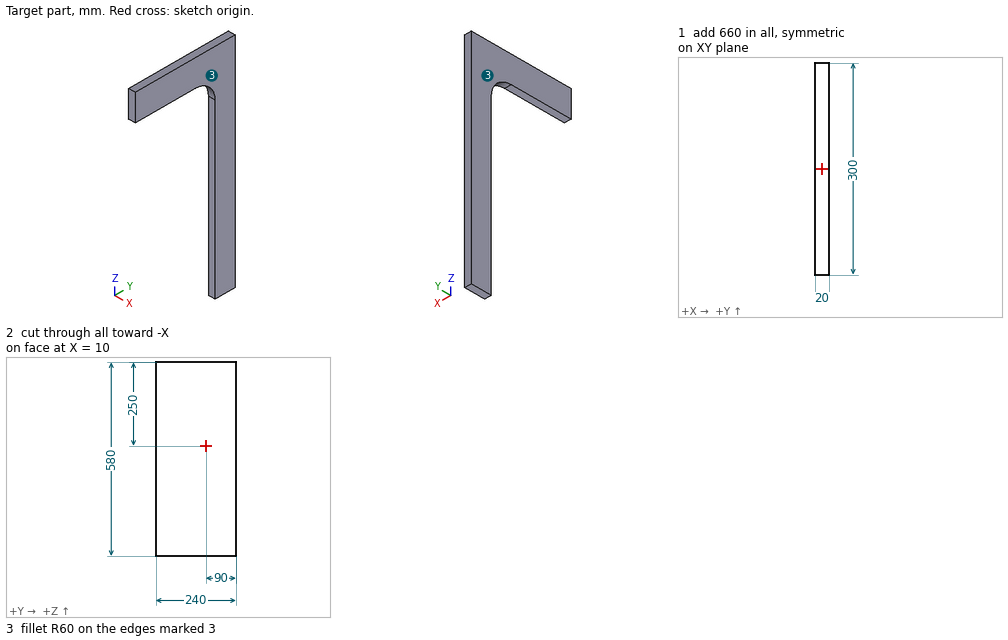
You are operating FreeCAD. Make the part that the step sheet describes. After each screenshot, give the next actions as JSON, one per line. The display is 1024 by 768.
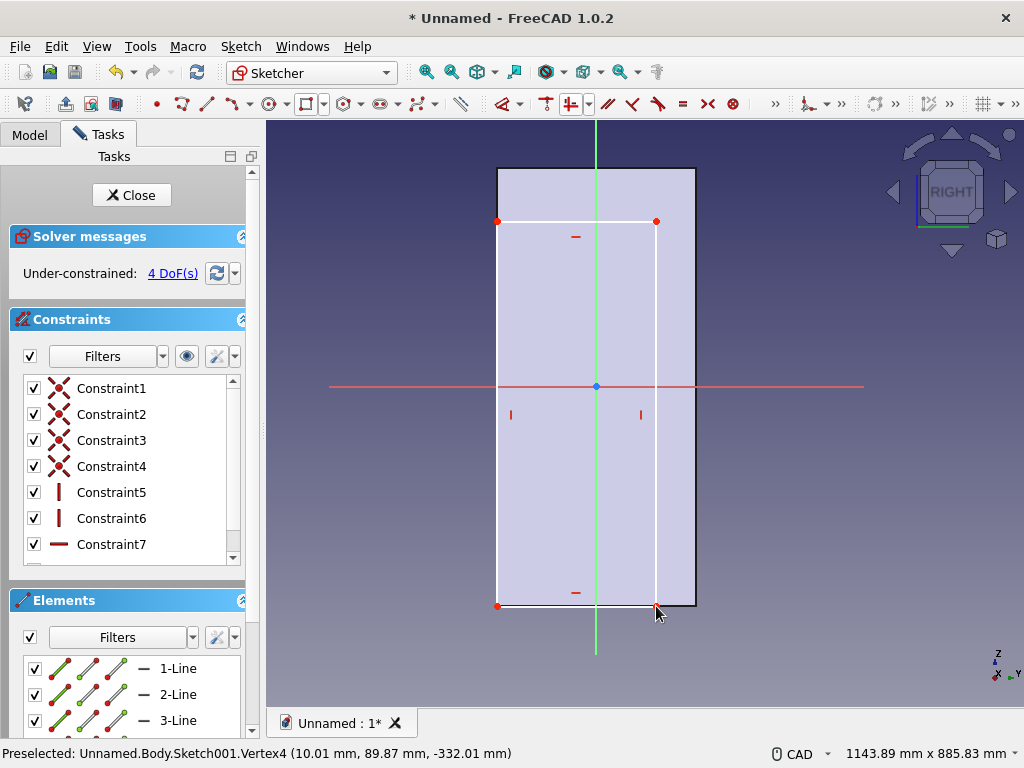
{"action": "key", "text": "d"}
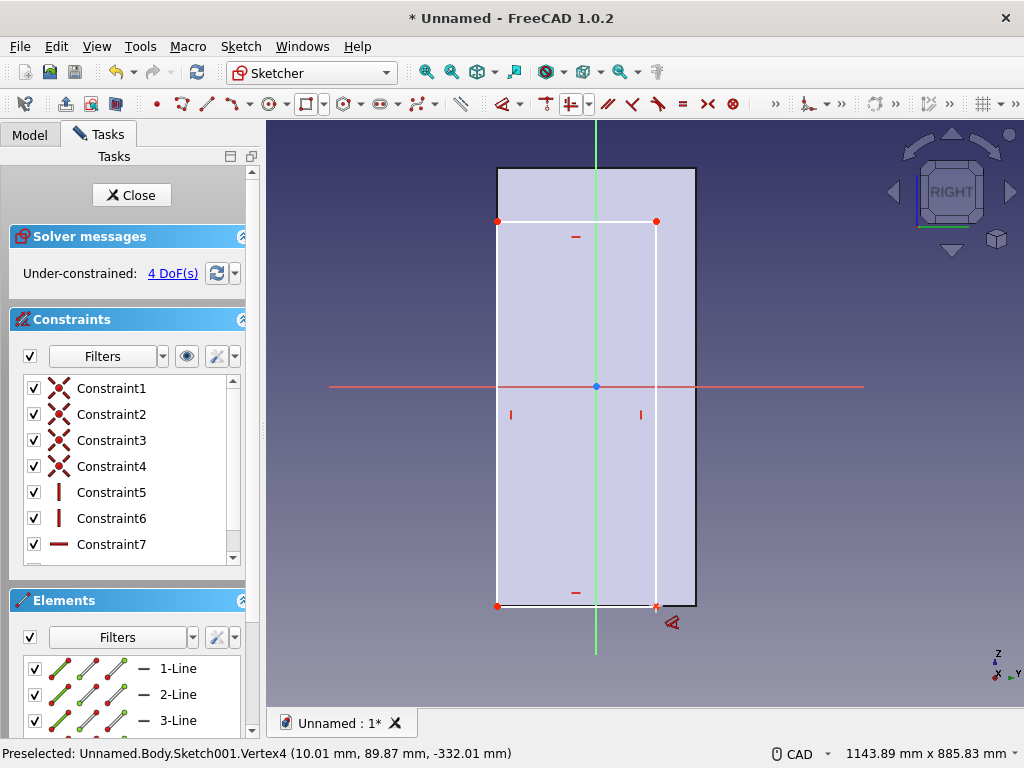
{"action": "left_click", "coordinate": [497, 337]}
{"action": "left_click", "coordinate": [463, 414]}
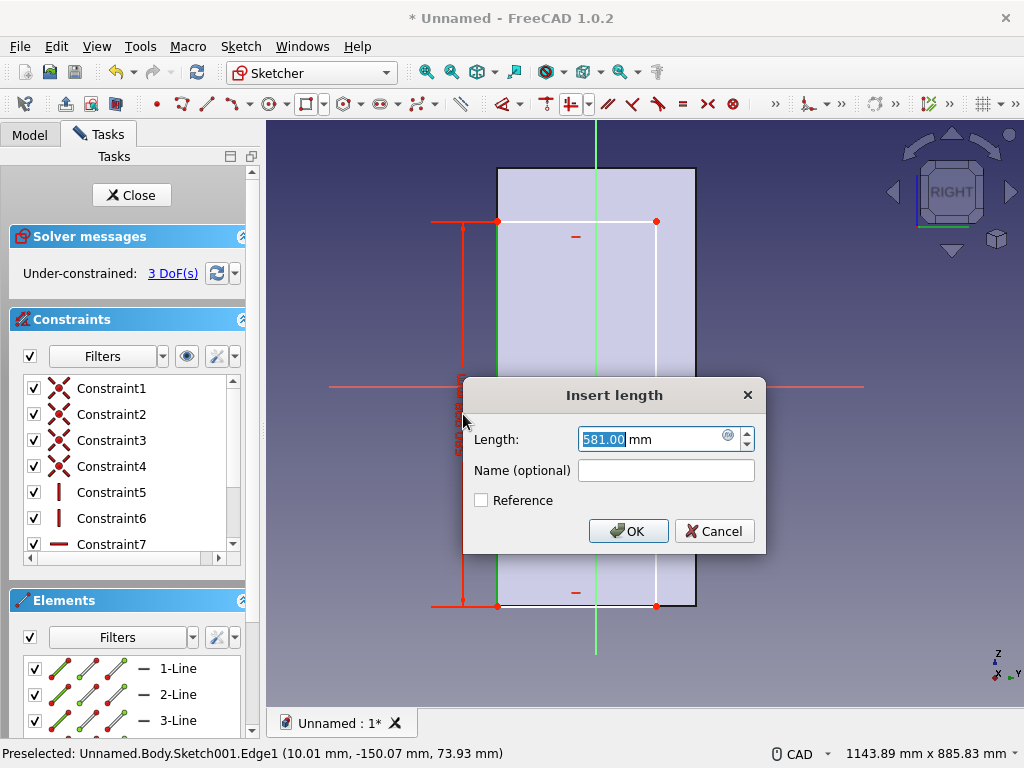
{"action": "type", "text": "580"}
{"action": "key", "text": "Return"}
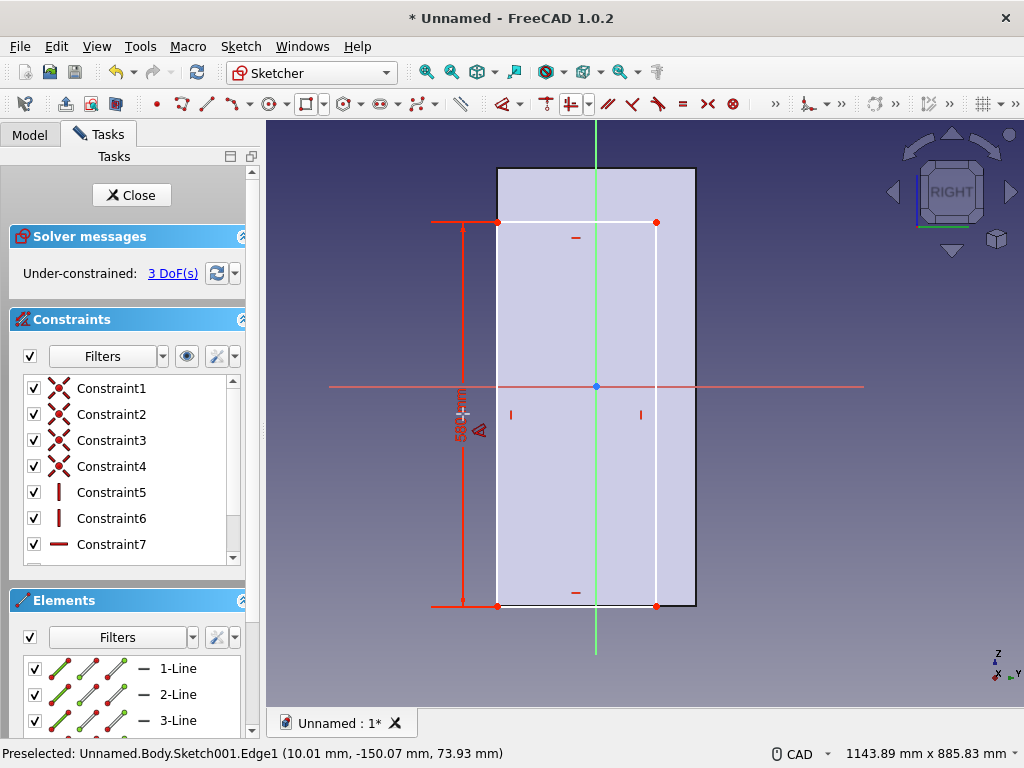
{"action": "left_click", "coordinate": [545, 607]}
{"action": "left_click", "coordinate": [576, 641]}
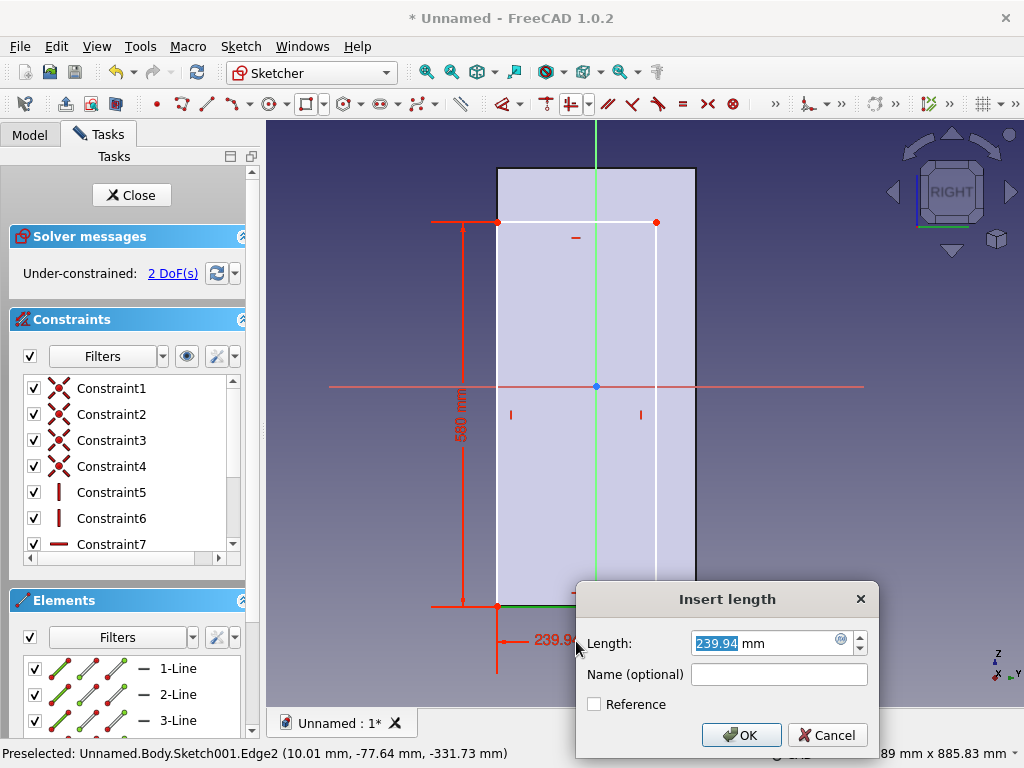
{"action": "type", "text": "240"}
{"action": "key", "text": "Return"}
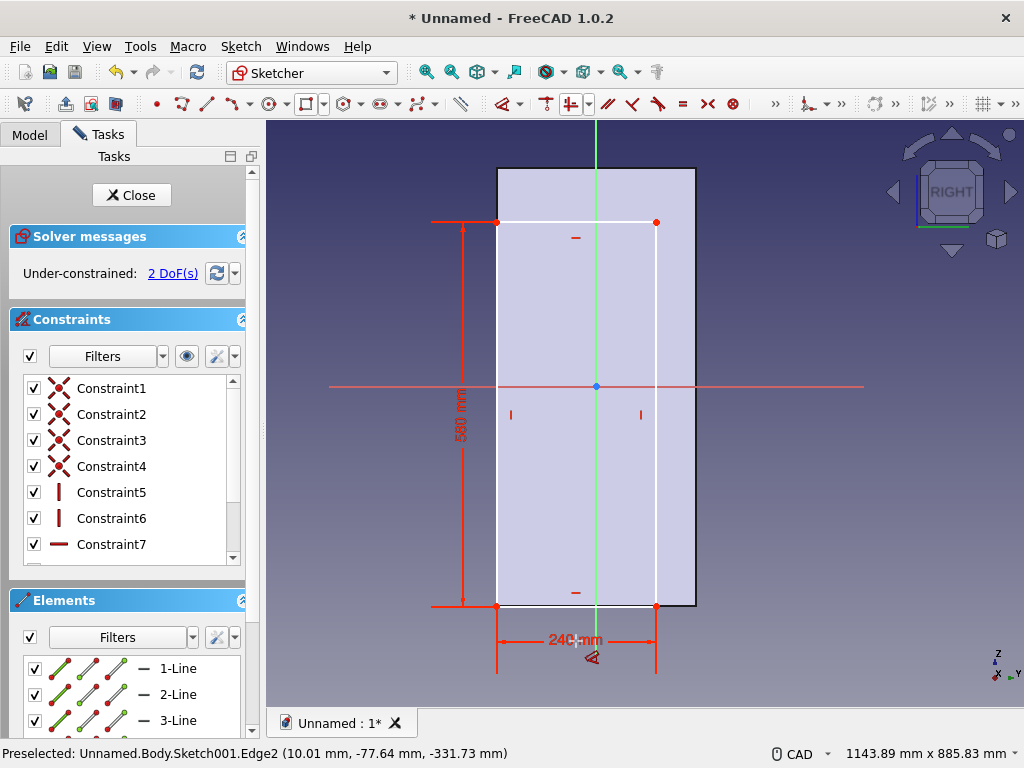
{"action": "left_click", "coordinate": [656, 607]}
{"action": "left_click", "coordinate": [647, 641]}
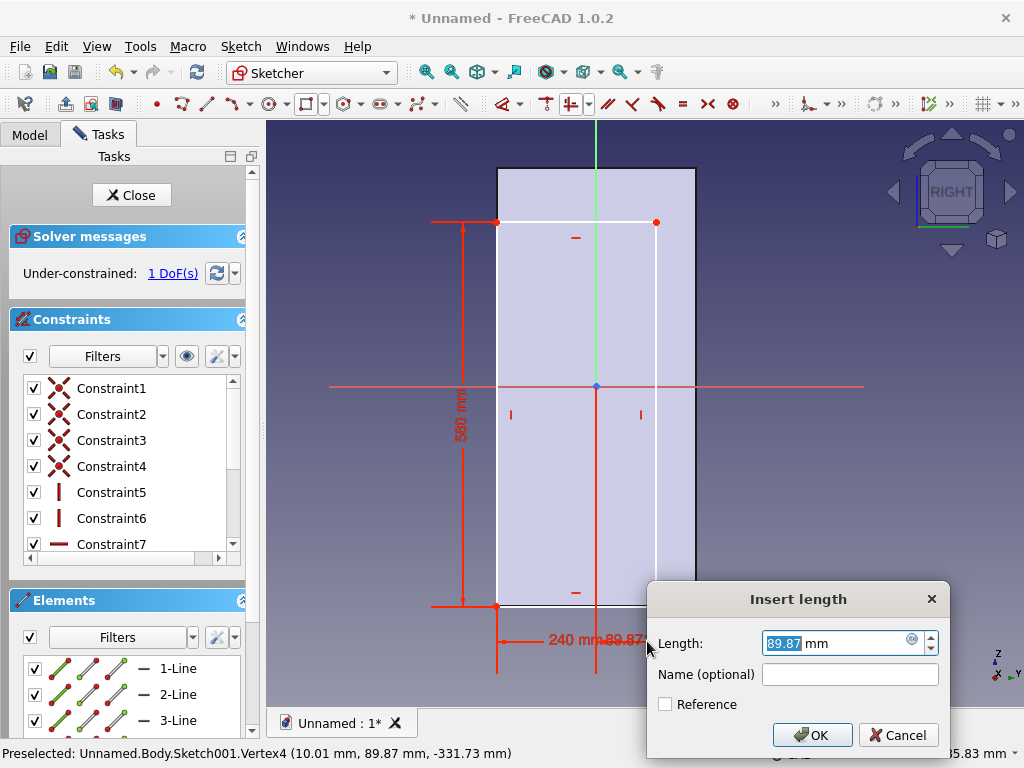
{"action": "type", "text": "90"}
{"action": "key", "text": "Return"}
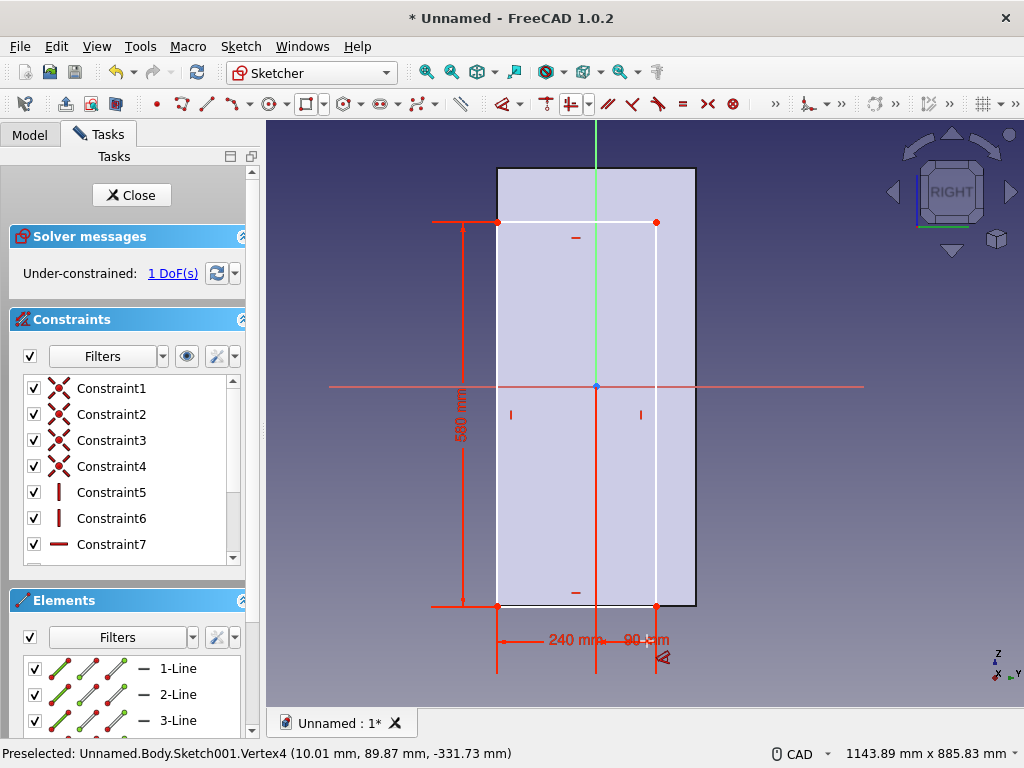
{"action": "left_click", "coordinate": [497, 222]}
{"action": "left_click", "coordinate": [463, 305]}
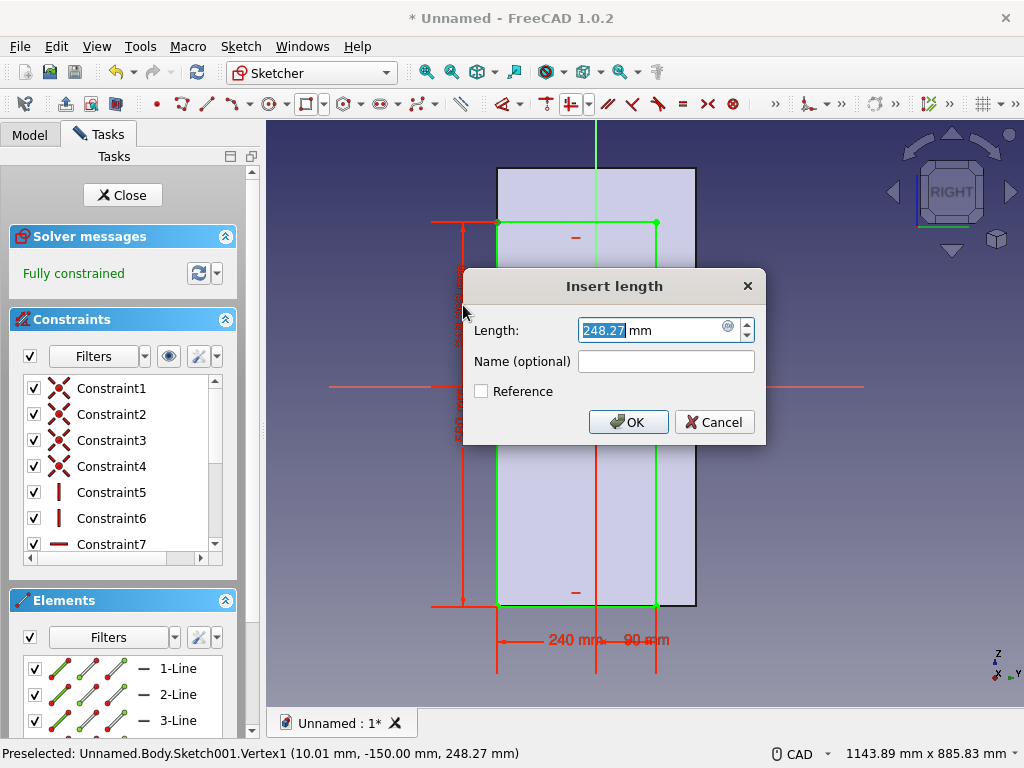
{"action": "type", "text": "250"}
{"action": "key", "text": "Return"}
{"action": "key", "text": "Escape"}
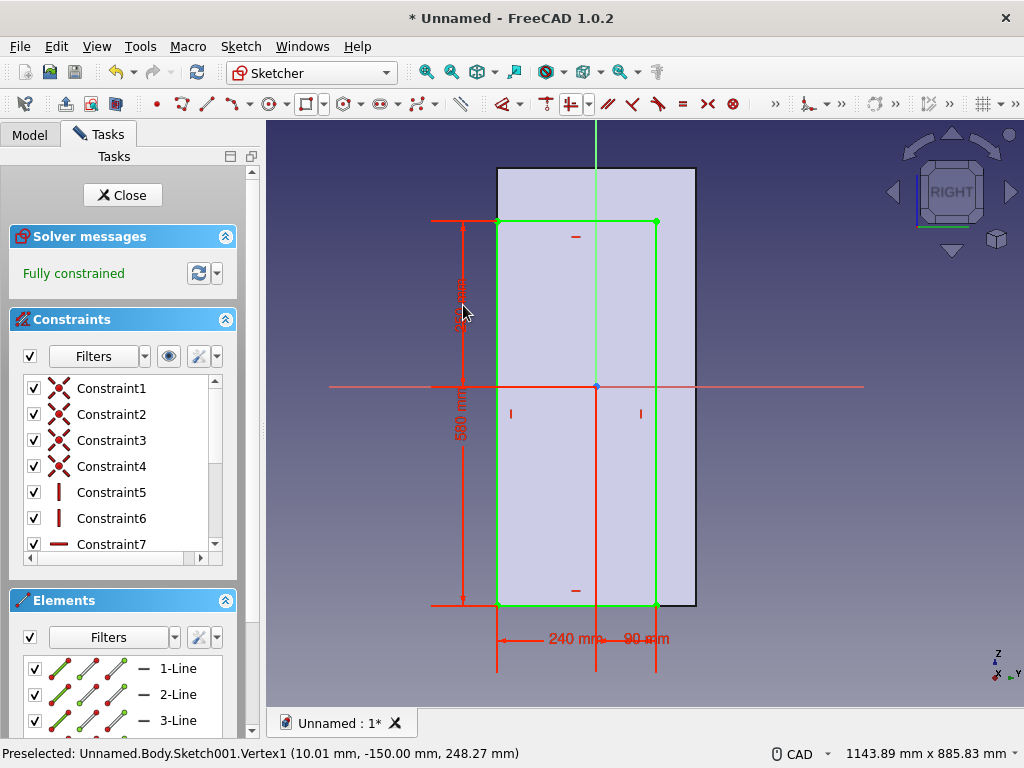
{"action": "left_click", "coordinate": [123, 195]}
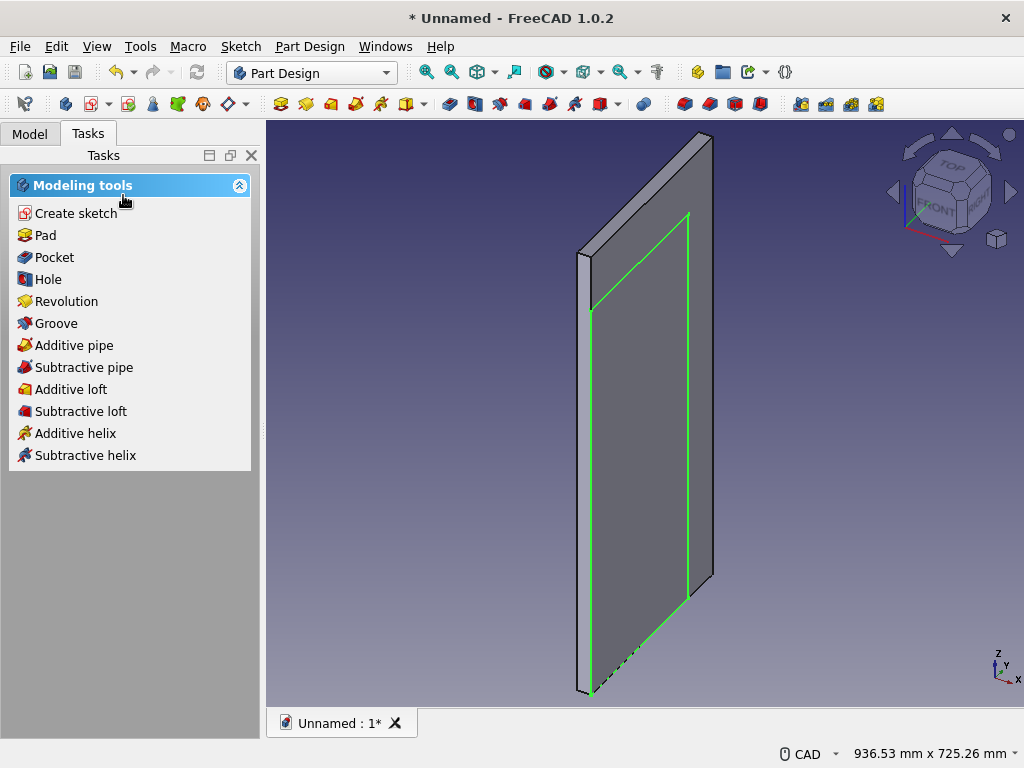
{"action": "left_click", "coordinate": [450, 104]}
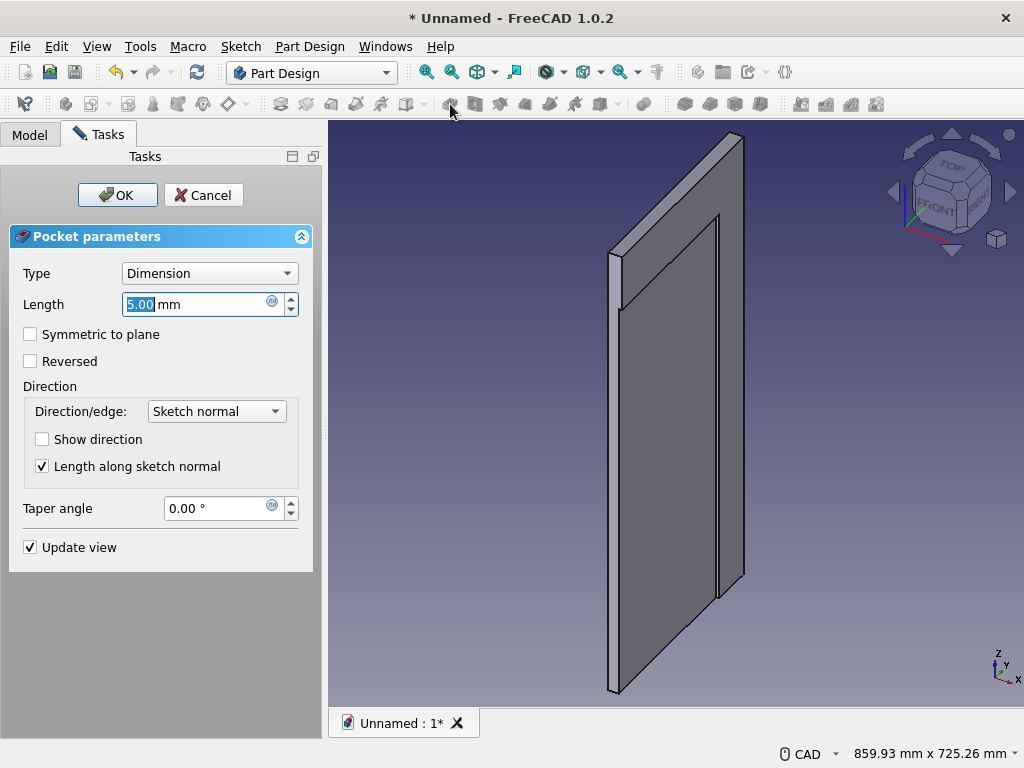
{"action": "left_click", "coordinate": [210, 274]}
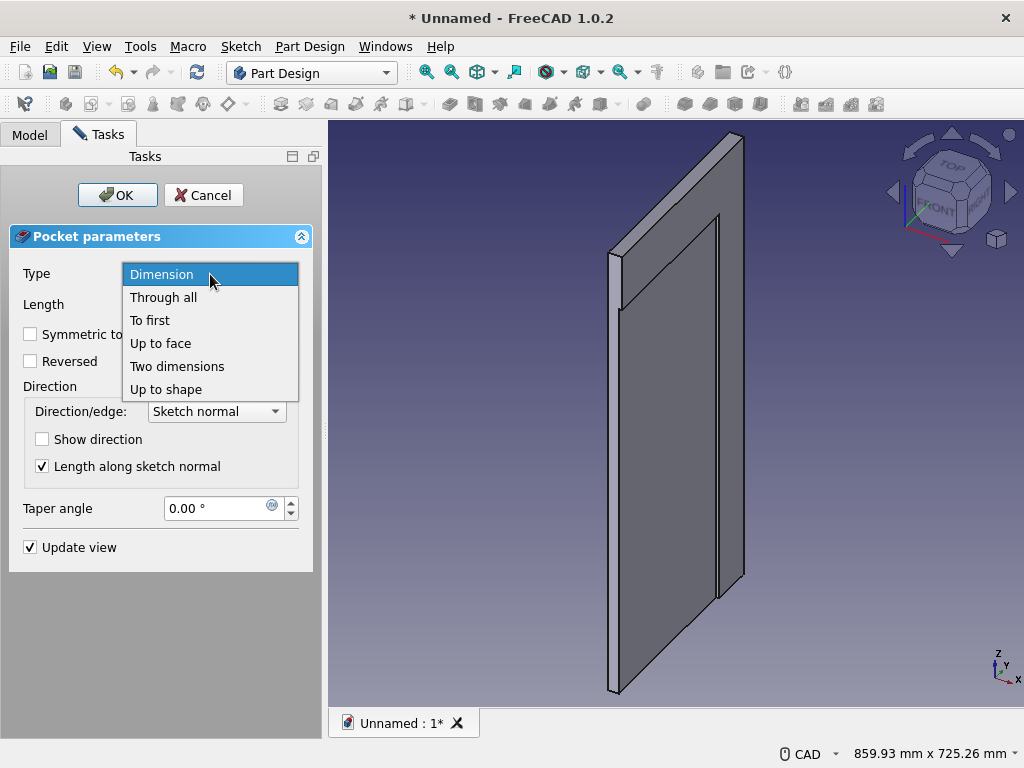
{"action": "left_click", "coordinate": [208, 298]}